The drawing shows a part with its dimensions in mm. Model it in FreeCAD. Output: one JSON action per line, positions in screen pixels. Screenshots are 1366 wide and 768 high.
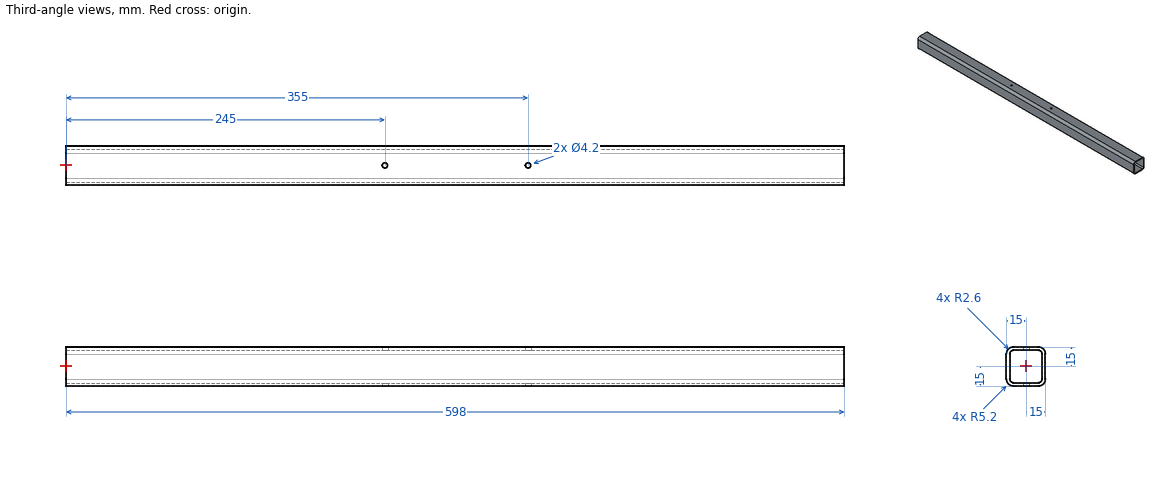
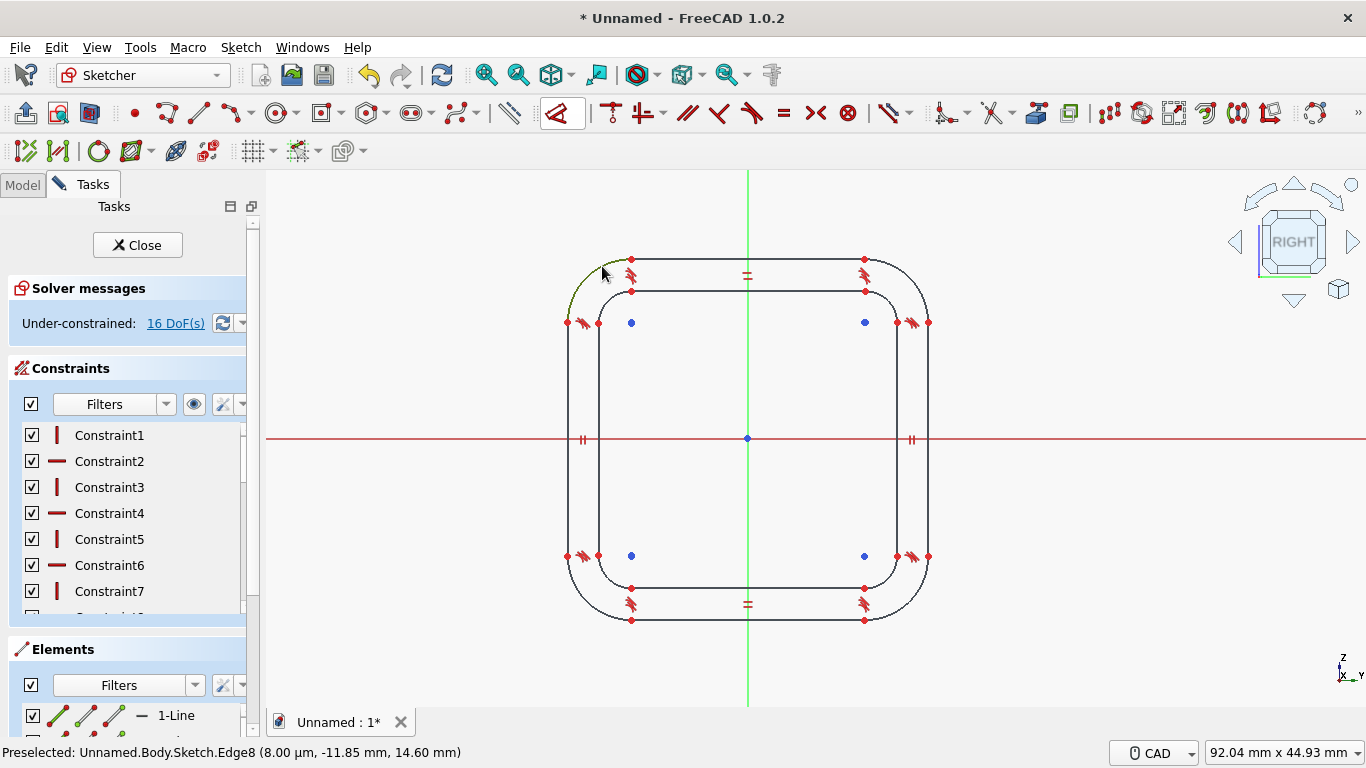
{"action": "left_click", "coordinate": [616, 295]}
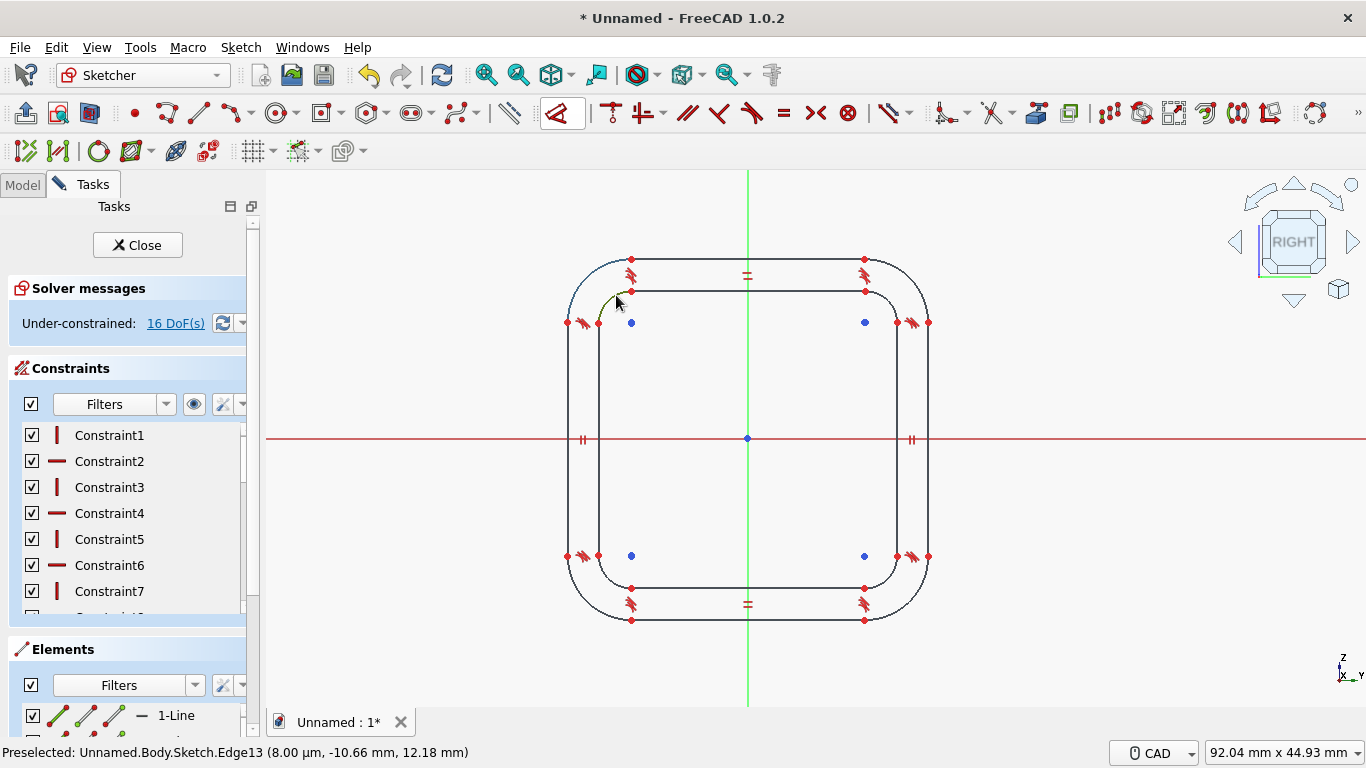
{"action": "left_click", "coordinate": [612, 114]}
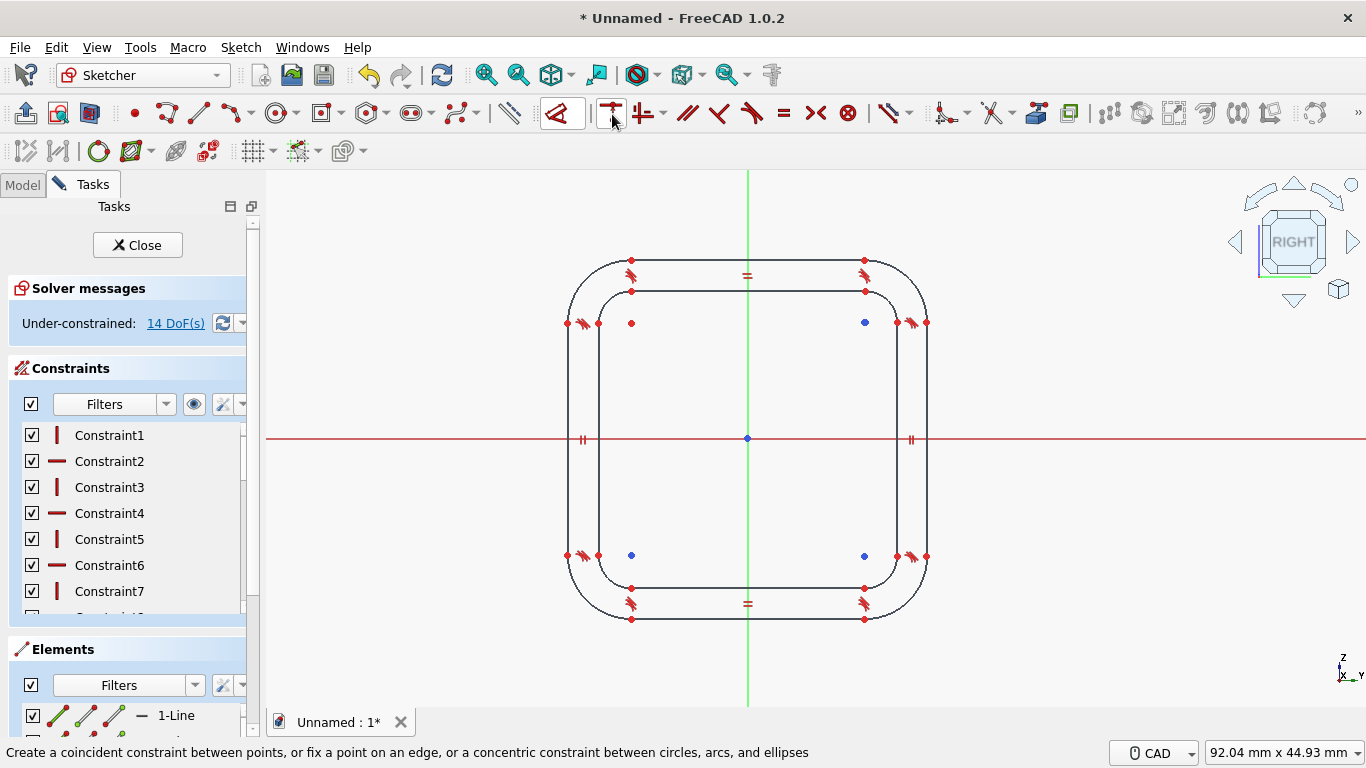
{"action": "left_click", "coordinate": [920, 294]}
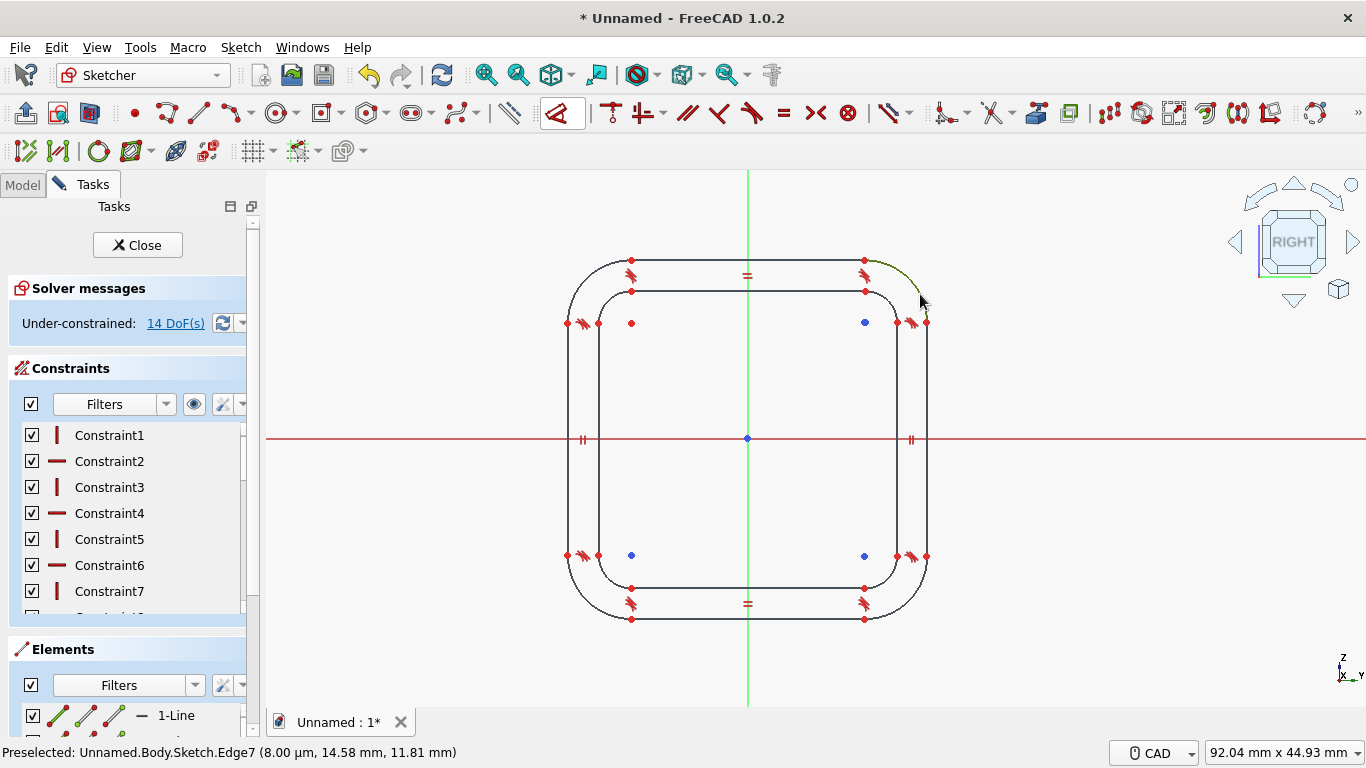
{"action": "left_click", "coordinate": [894, 309]}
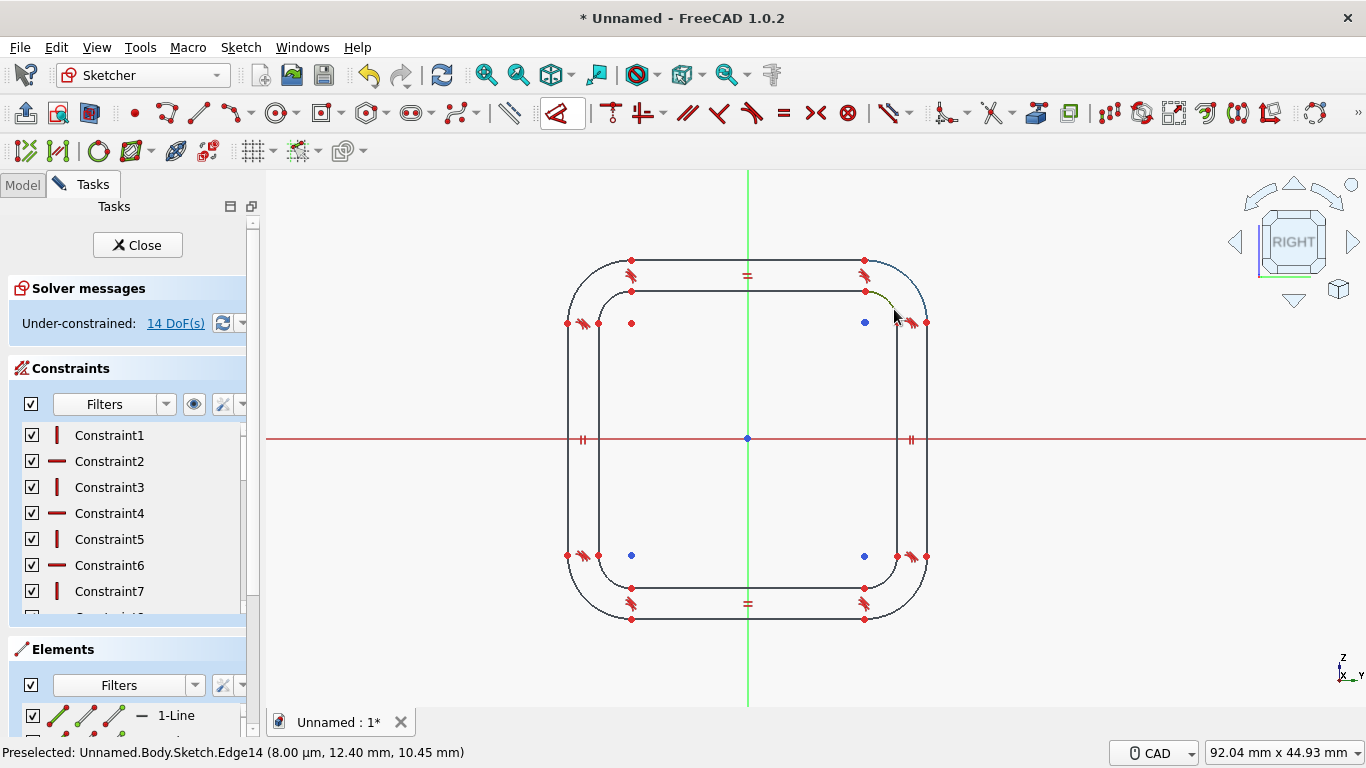
{"action": "key", "text": "c"}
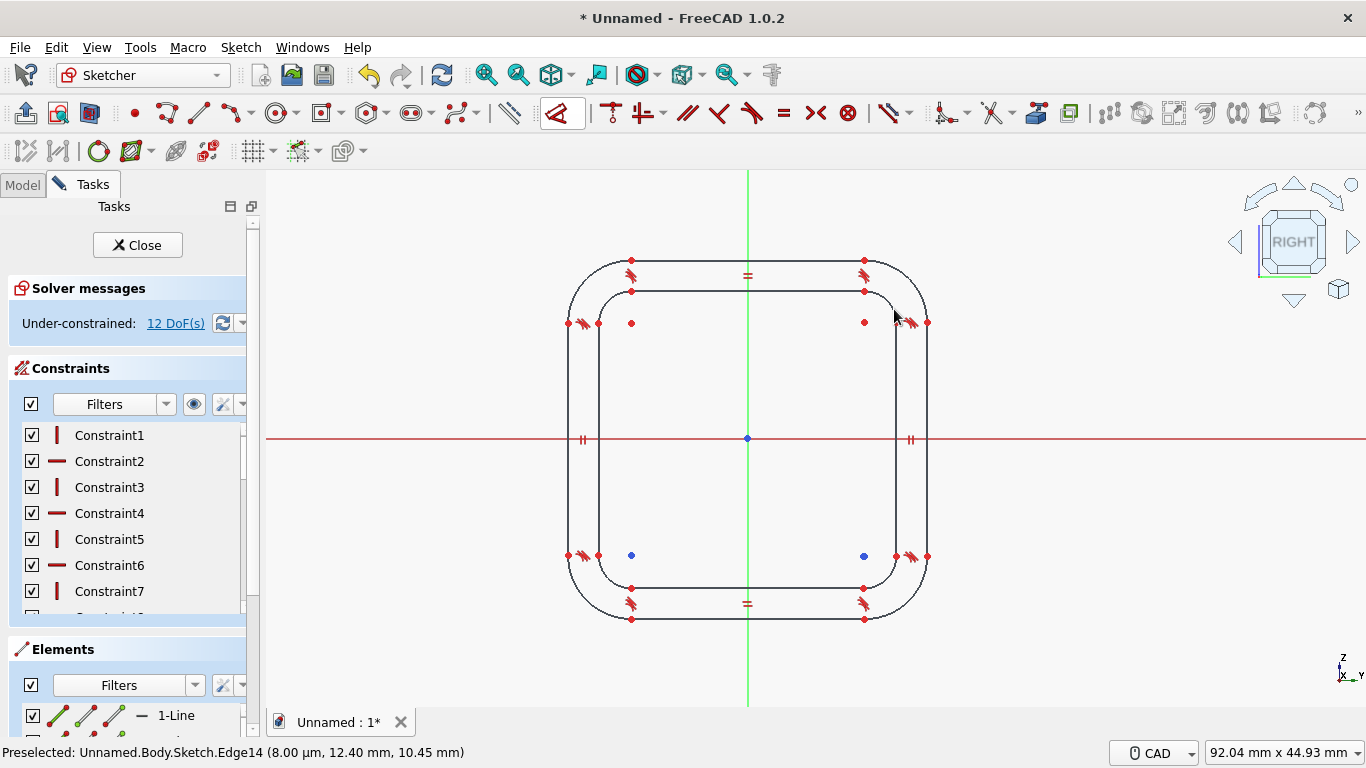
{"action": "left_click", "coordinate": [893, 612]}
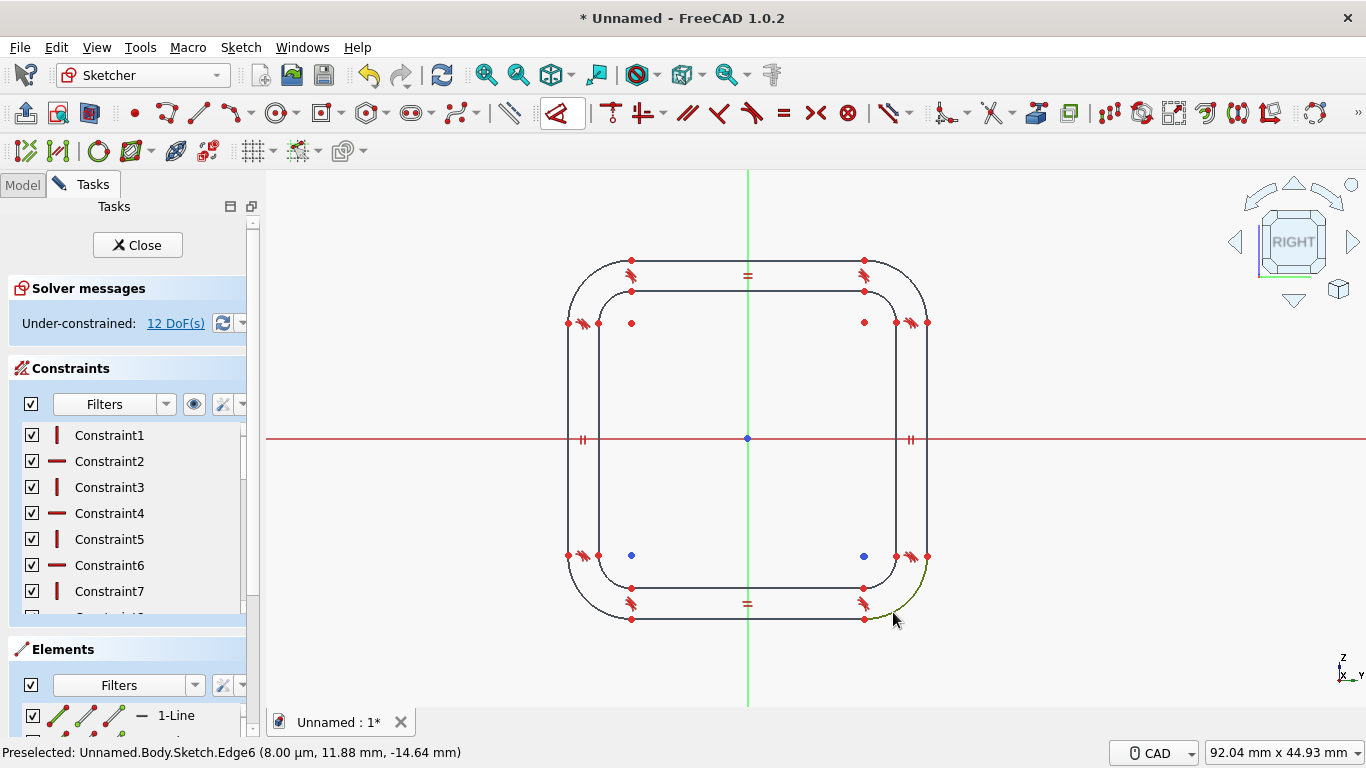
{"action": "left_click", "coordinate": [879, 585]}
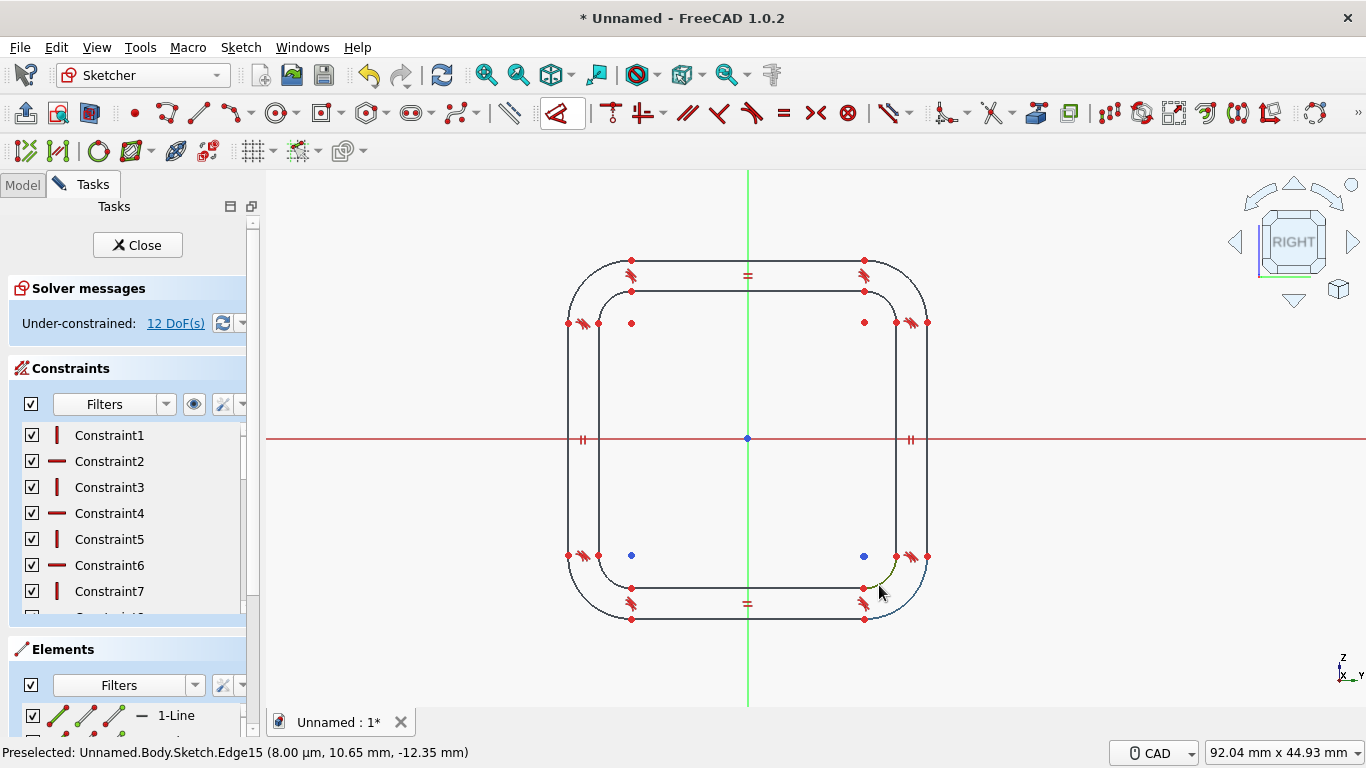
{"action": "left_click", "coordinate": [612, 114]}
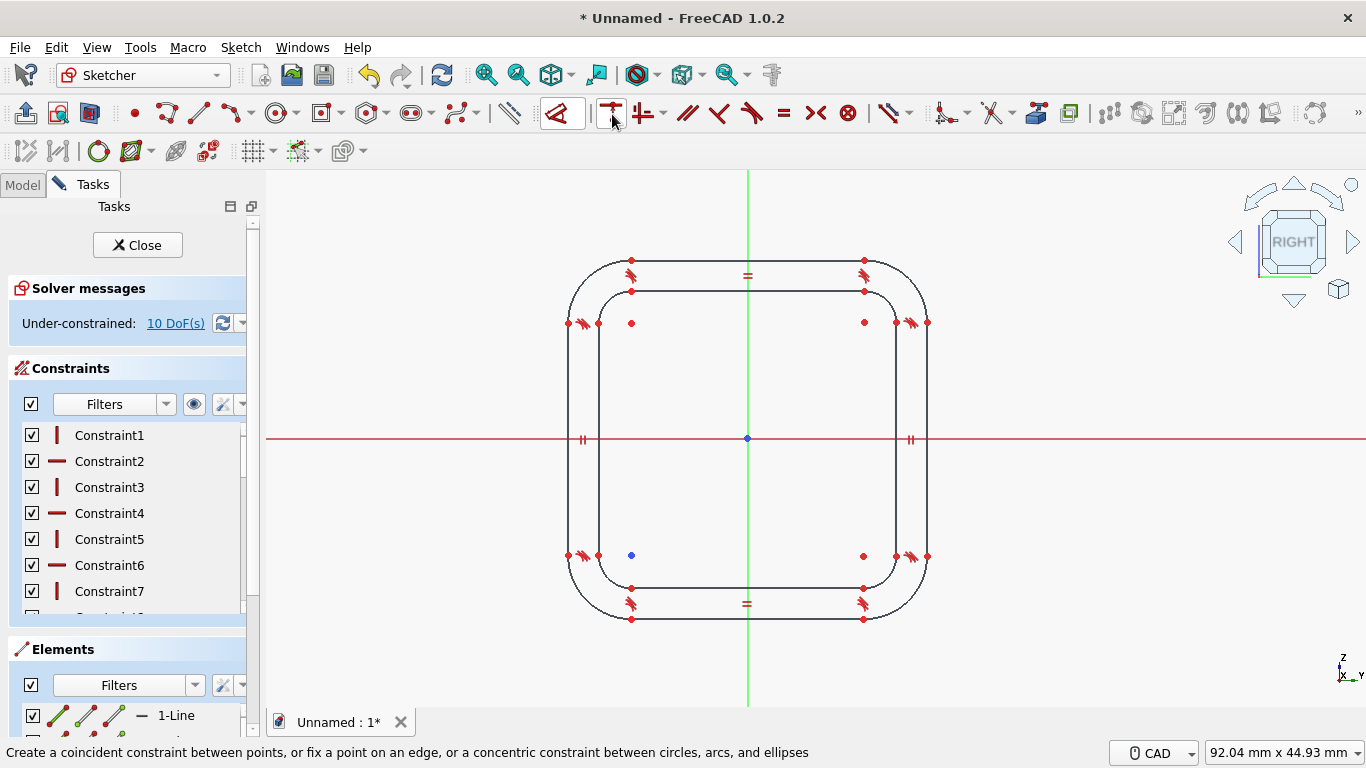
{"action": "left_click", "coordinate": [575, 584]}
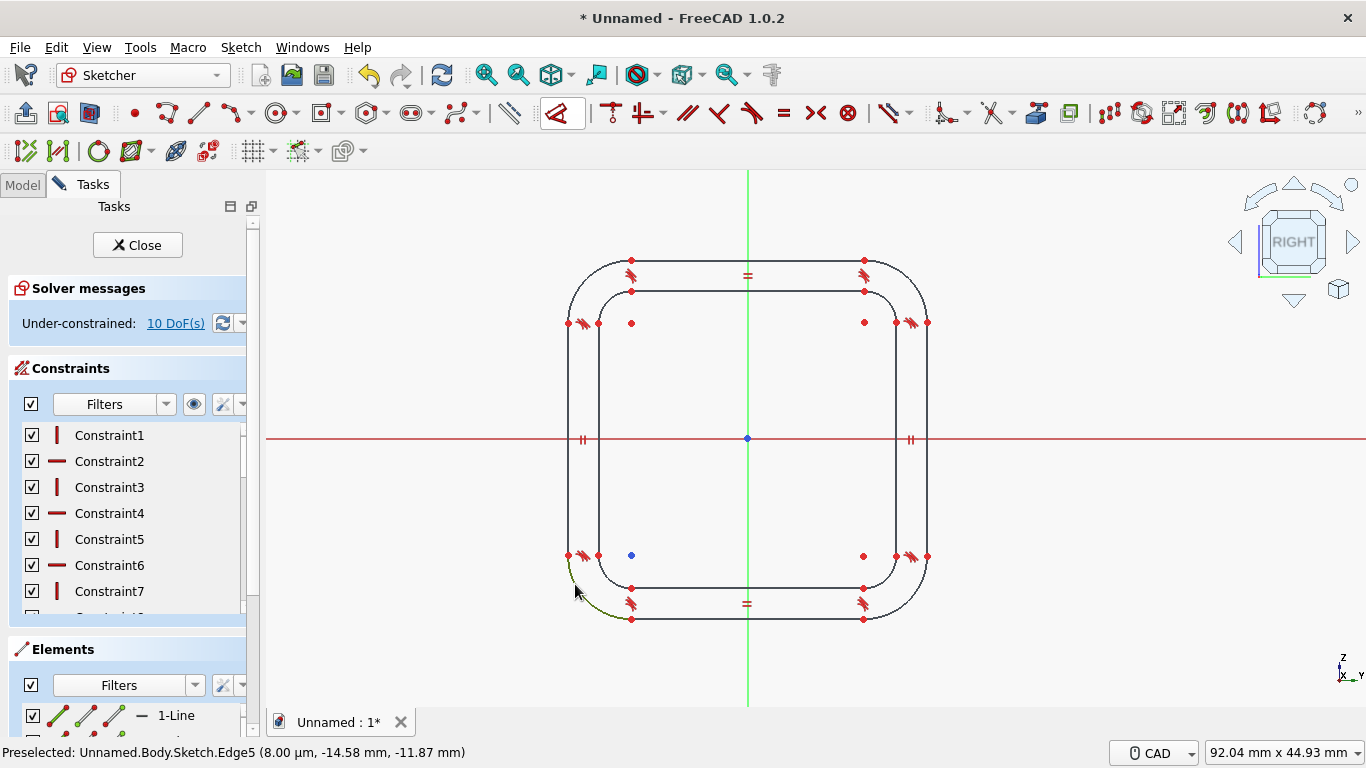
{"action": "left_click", "coordinate": [893, 612]}